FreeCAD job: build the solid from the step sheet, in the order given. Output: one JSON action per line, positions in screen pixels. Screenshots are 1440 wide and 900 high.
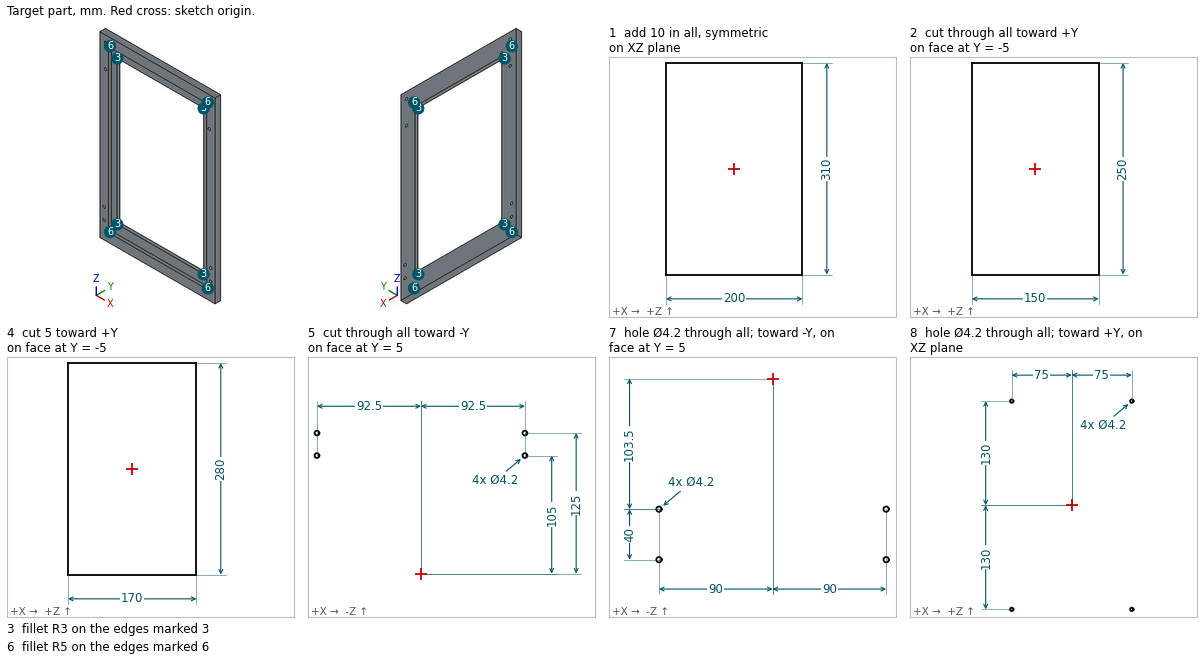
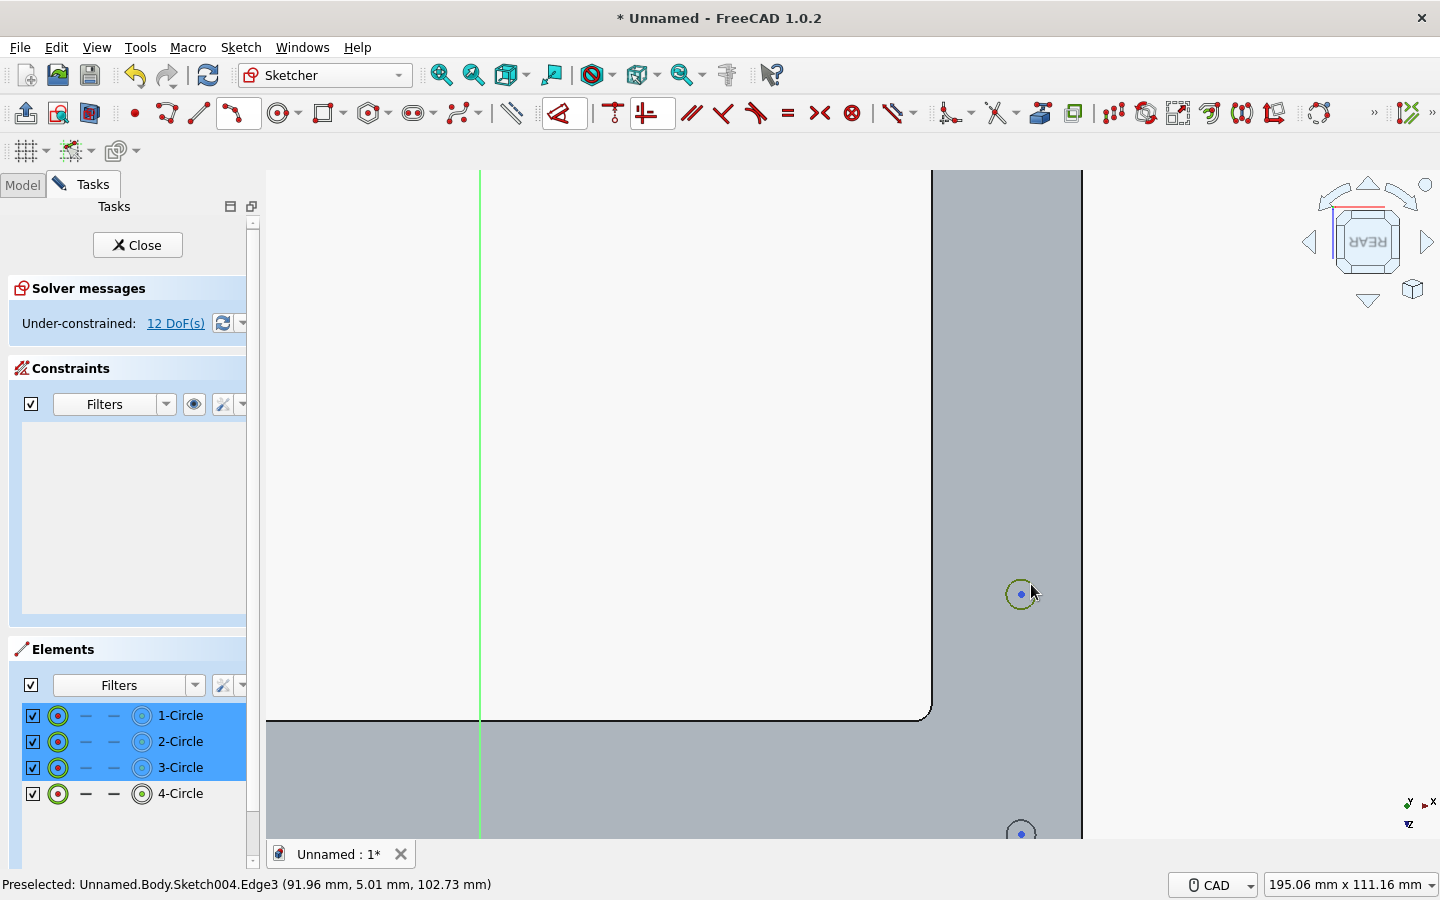
{"action": "scroll", "coordinate": [1033, 584], "scroll_direction": "down", "scroll_amount": 4}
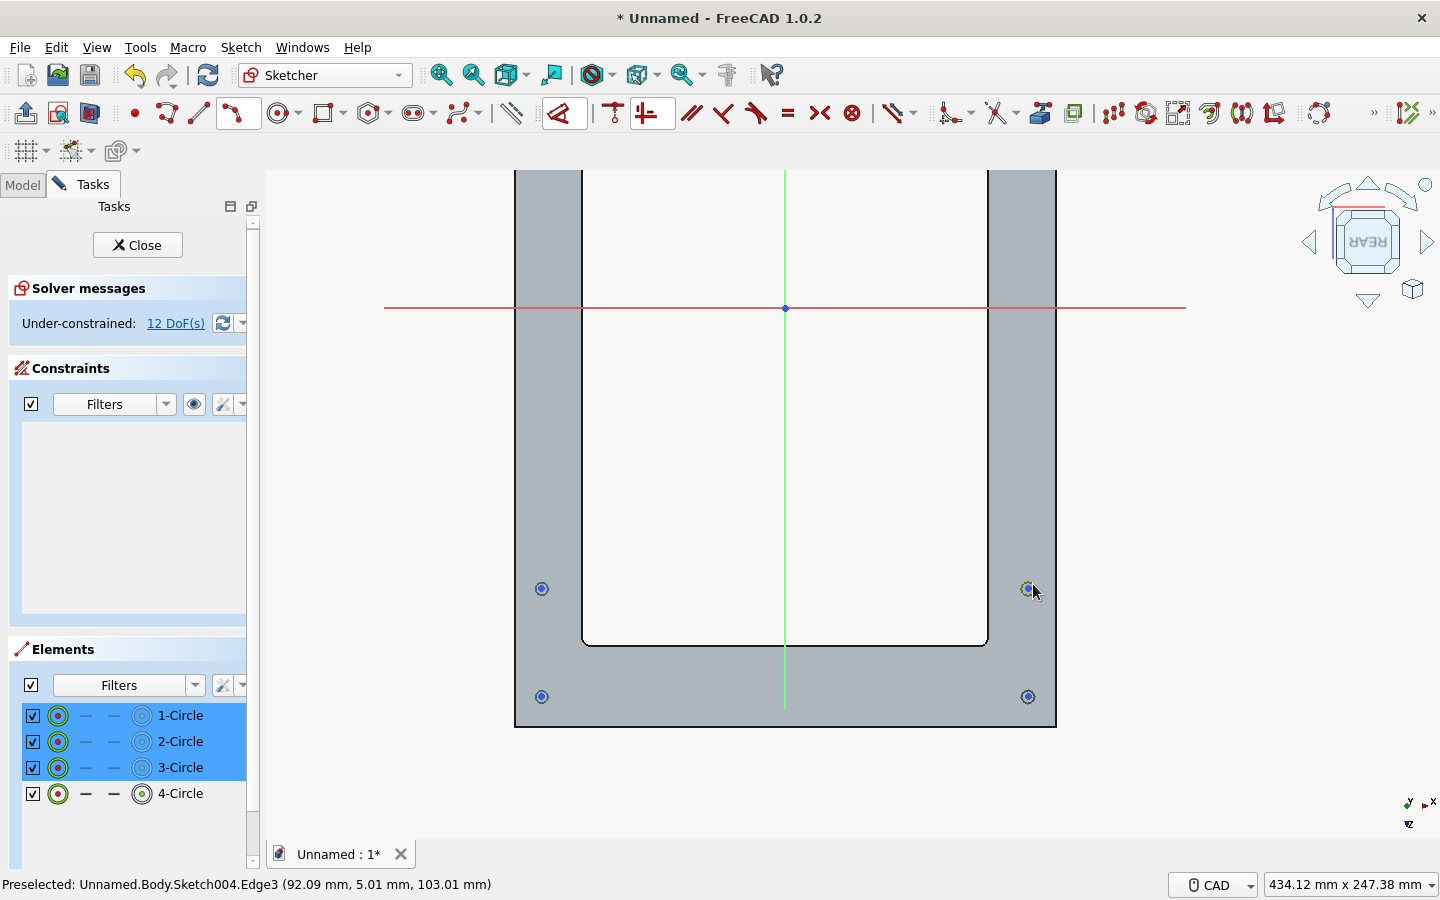
{"action": "scroll", "coordinate": [1033, 692], "scroll_direction": "up", "scroll_amount": 4}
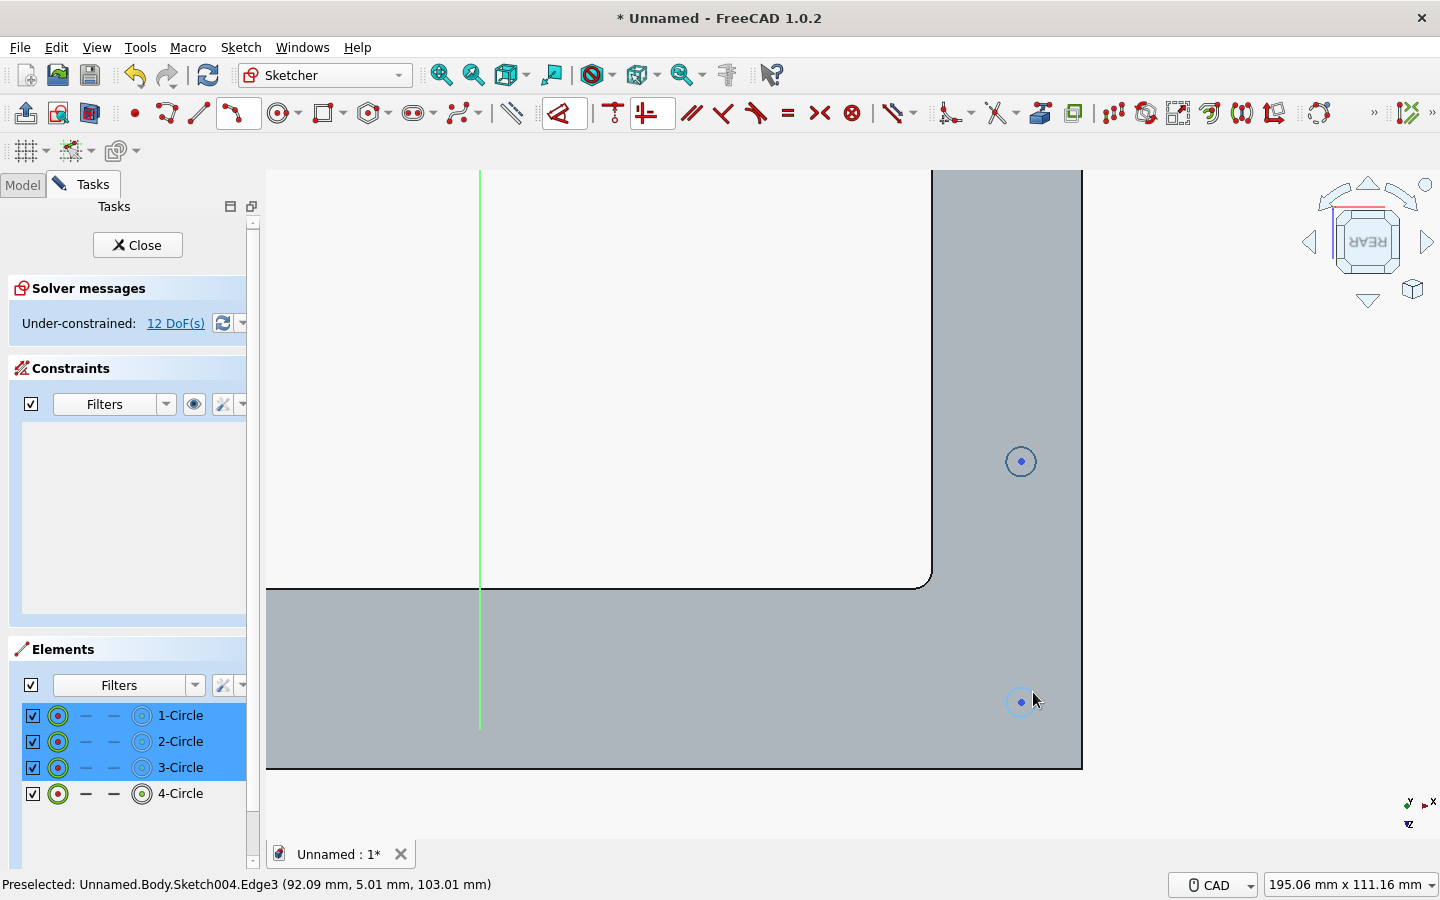
{"action": "left_click", "coordinate": [1031, 692]}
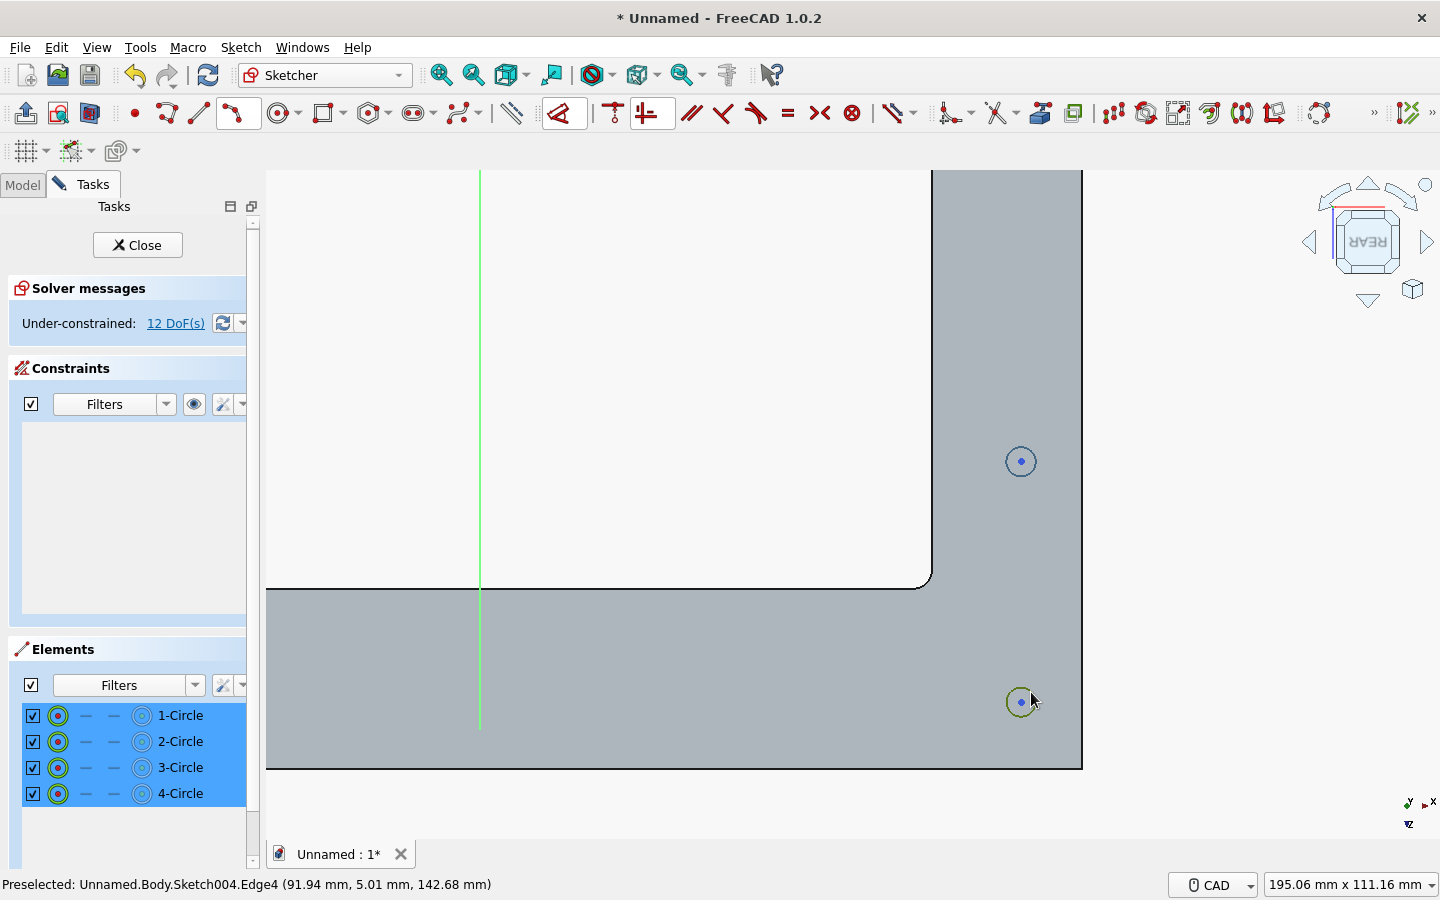
{"action": "left_click", "coordinate": [788, 114]}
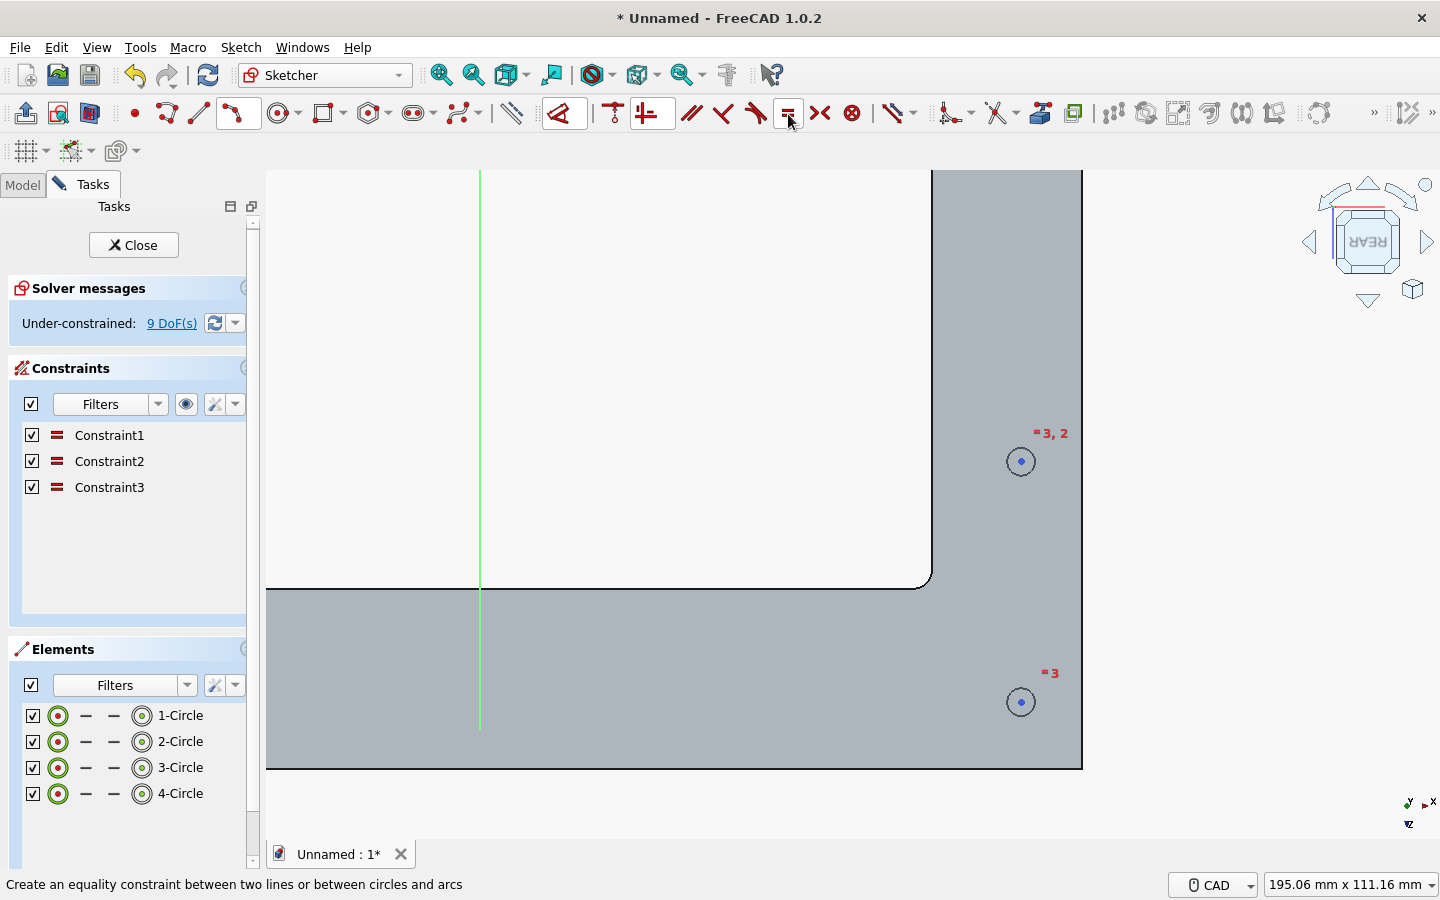
{"action": "scroll", "coordinate": [1033, 692], "scroll_direction": "down", "scroll_amount": 4}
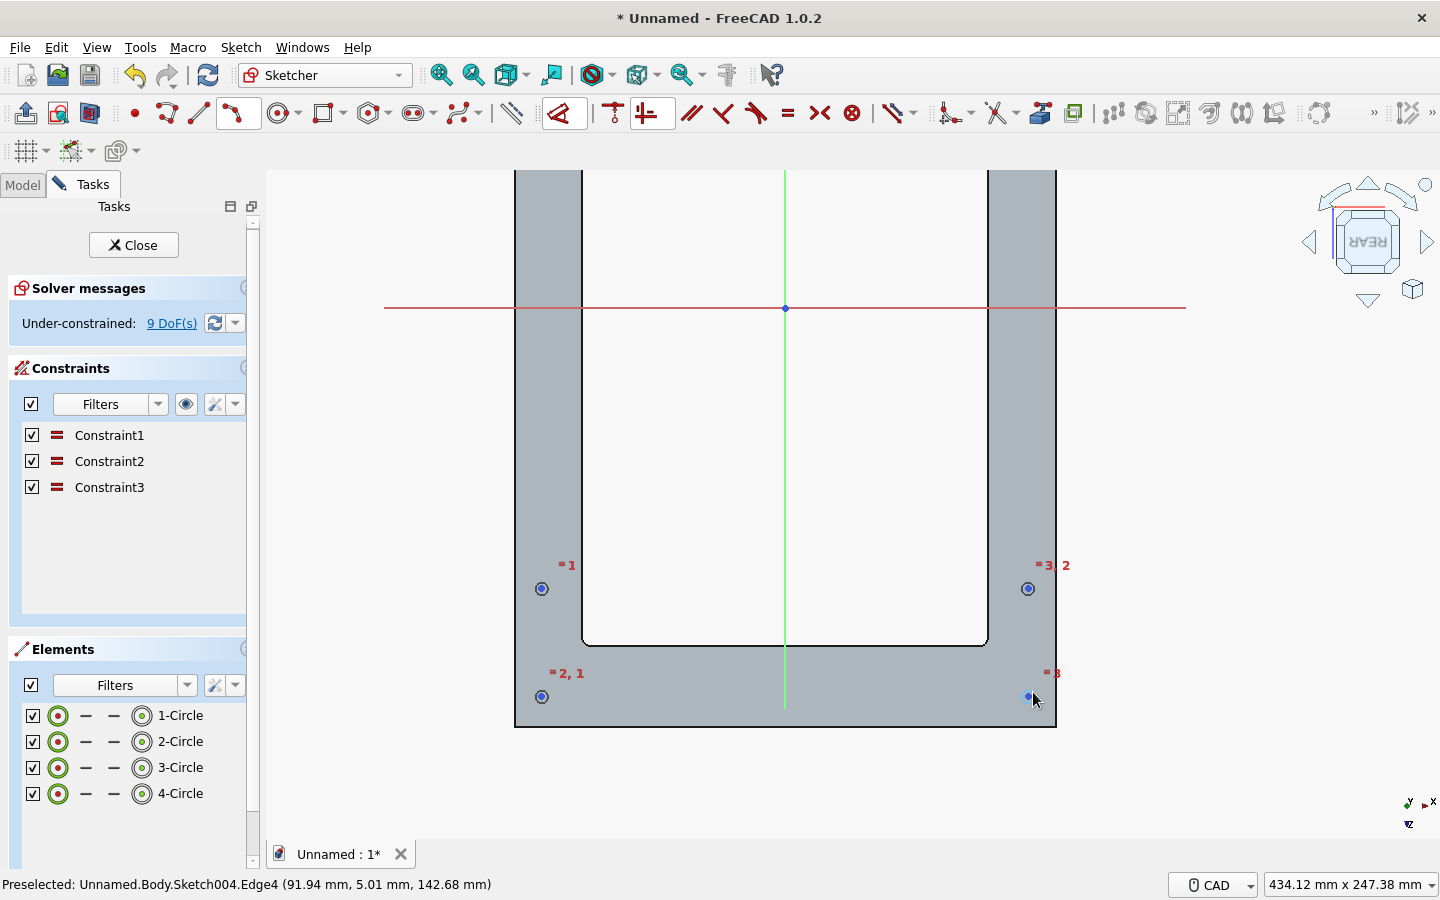
{"action": "left_click", "coordinate": [542, 589]}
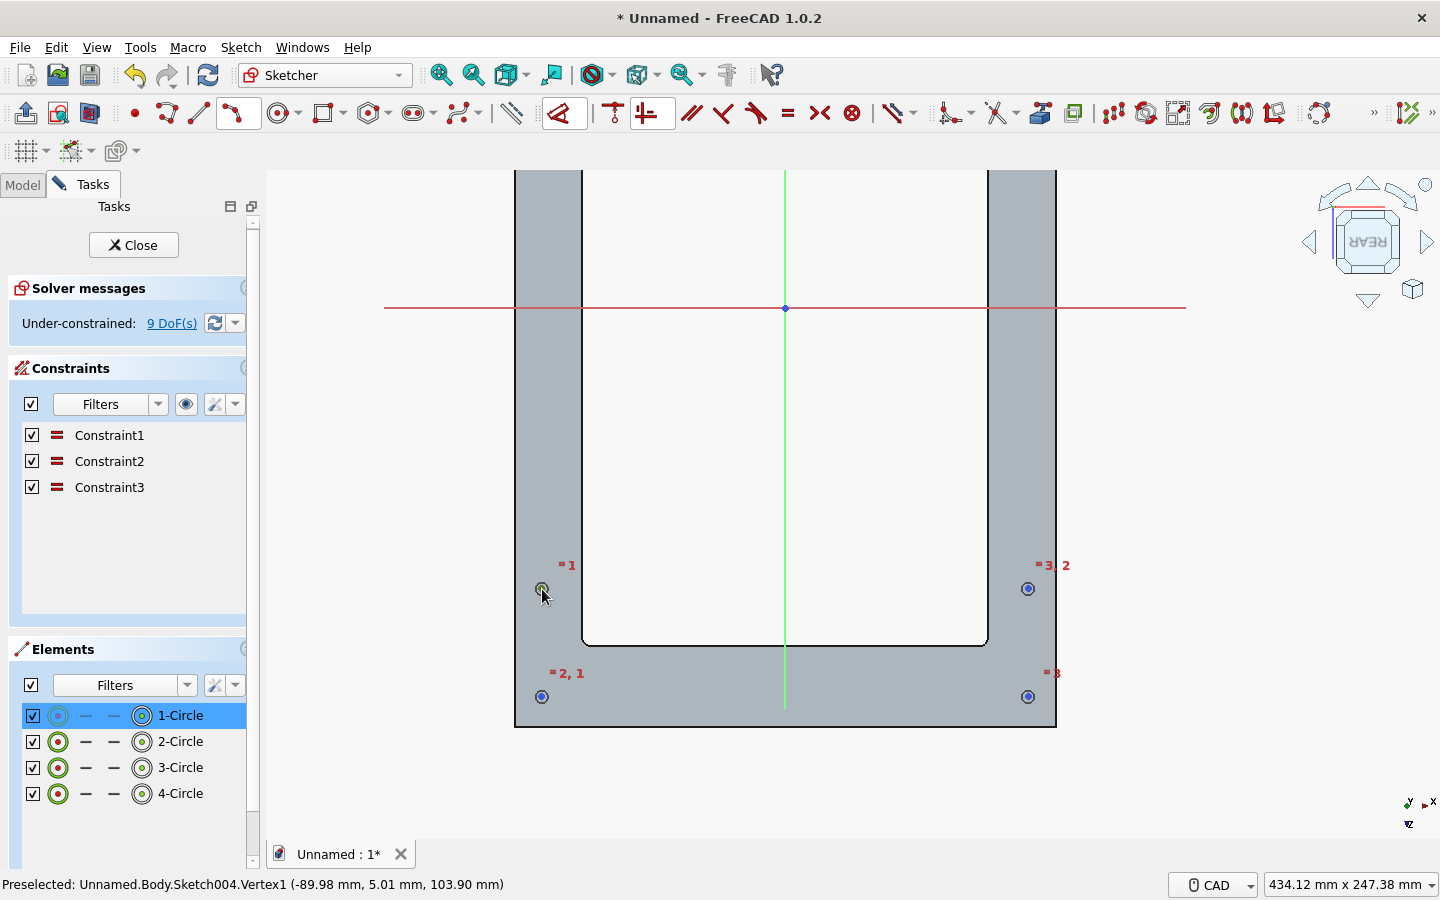
{"action": "left_click", "coordinate": [542, 697]}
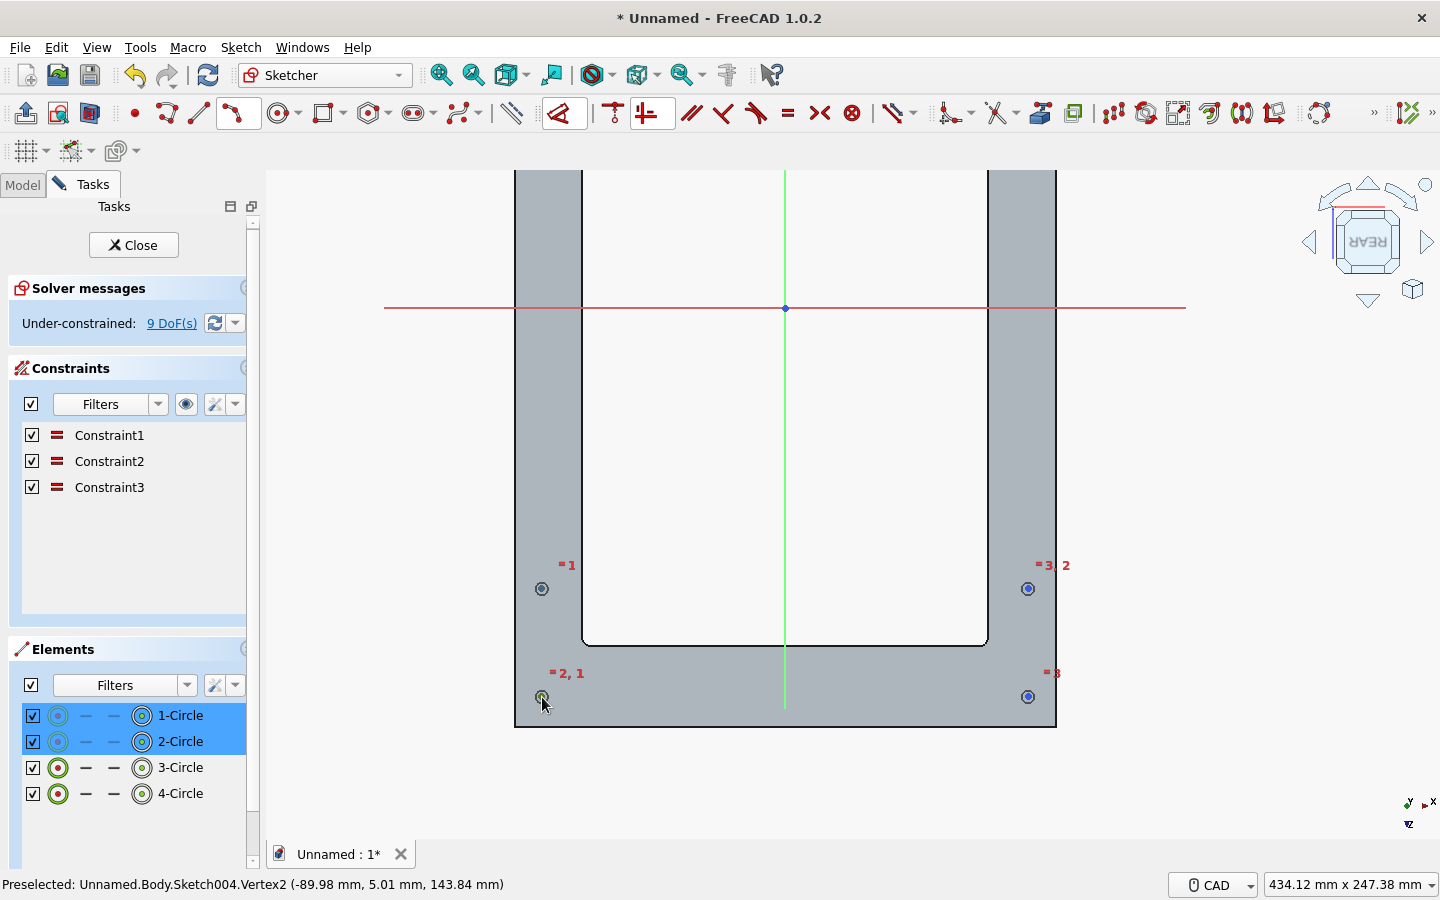
{"action": "key", "text": "v"}